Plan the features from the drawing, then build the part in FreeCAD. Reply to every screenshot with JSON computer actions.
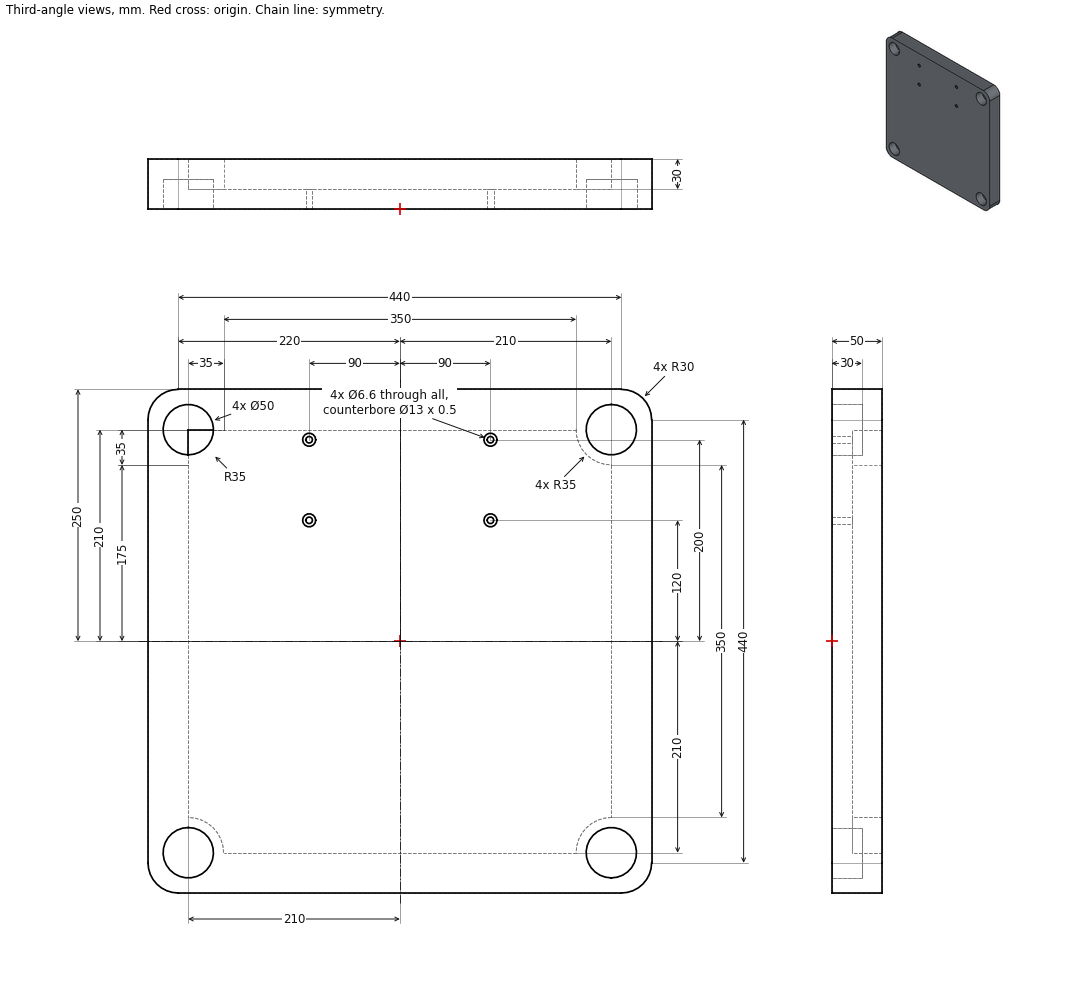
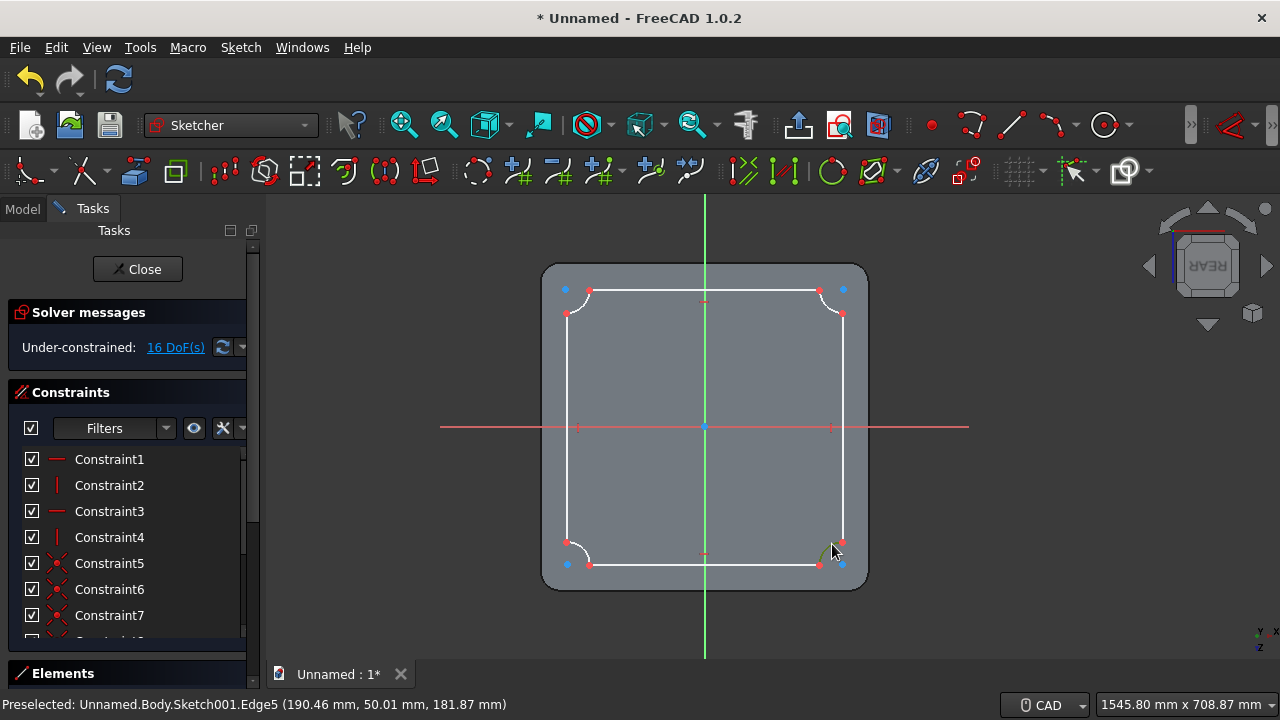
{"action": "scroll", "coordinate": [823, 301], "scroll_direction": "up", "scroll_amount": 2}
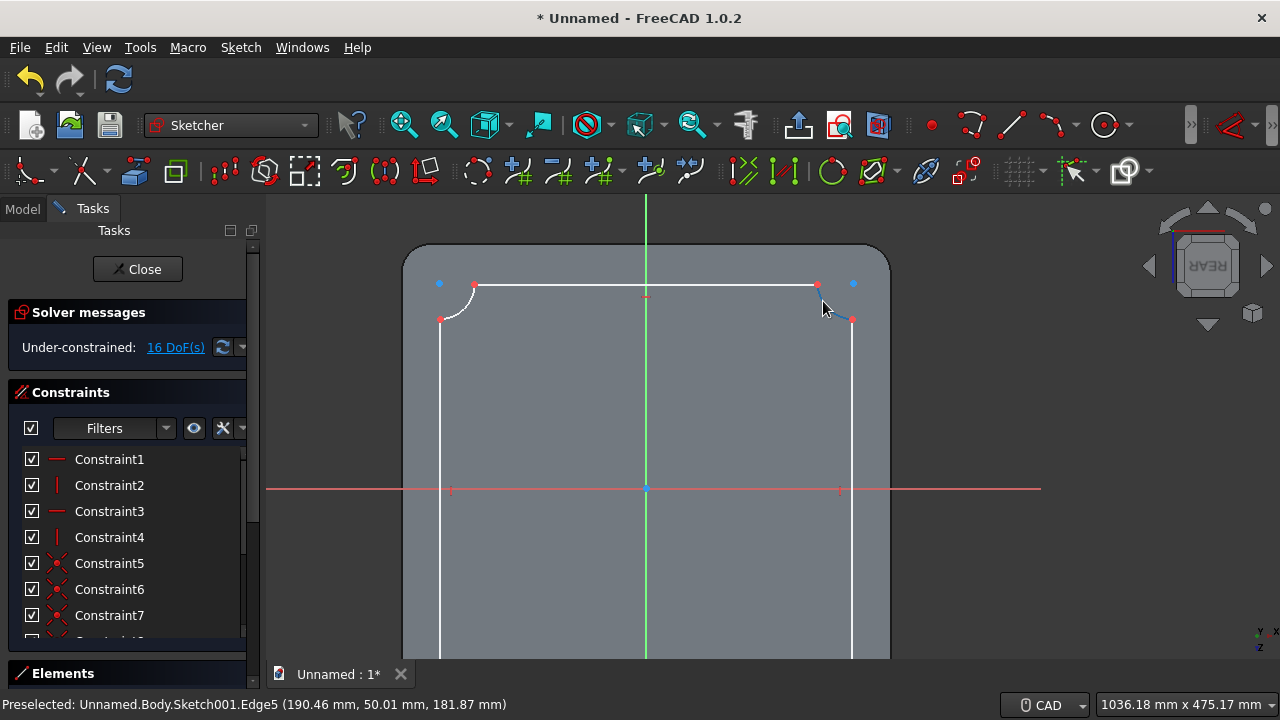
{"action": "left_click", "coordinate": [822, 300]}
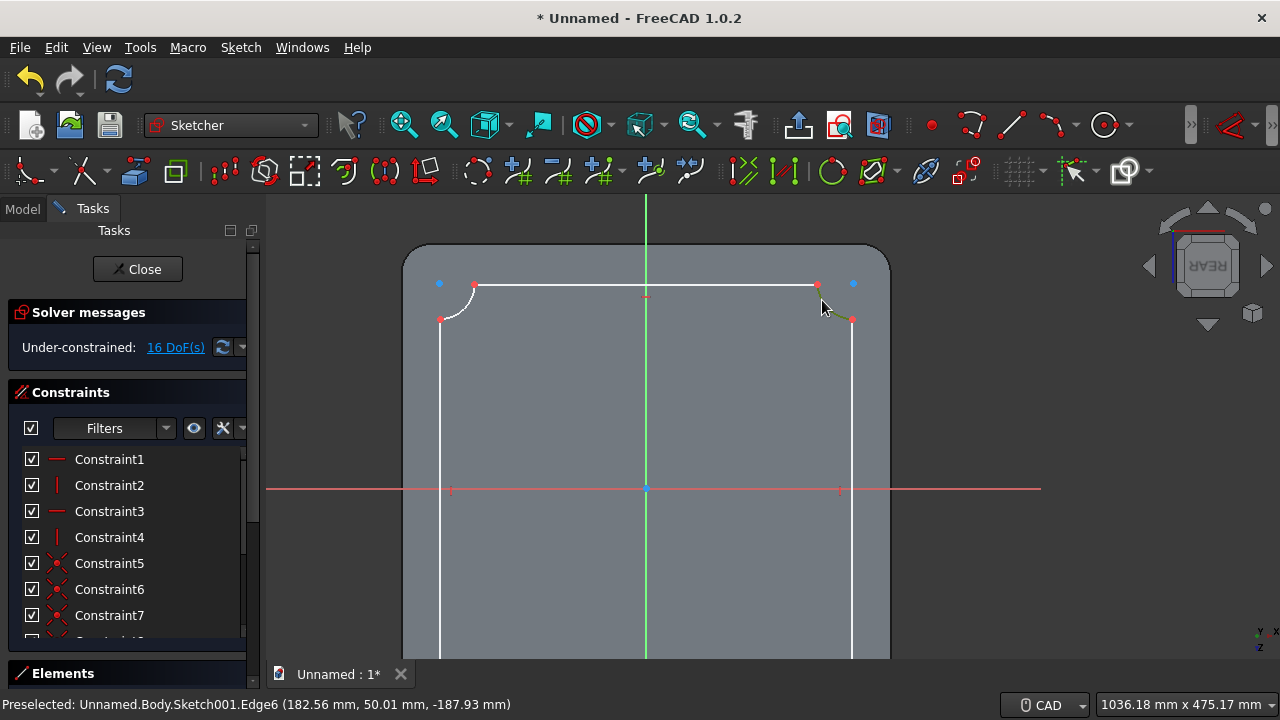
{"action": "left_click", "coordinate": [456, 315]}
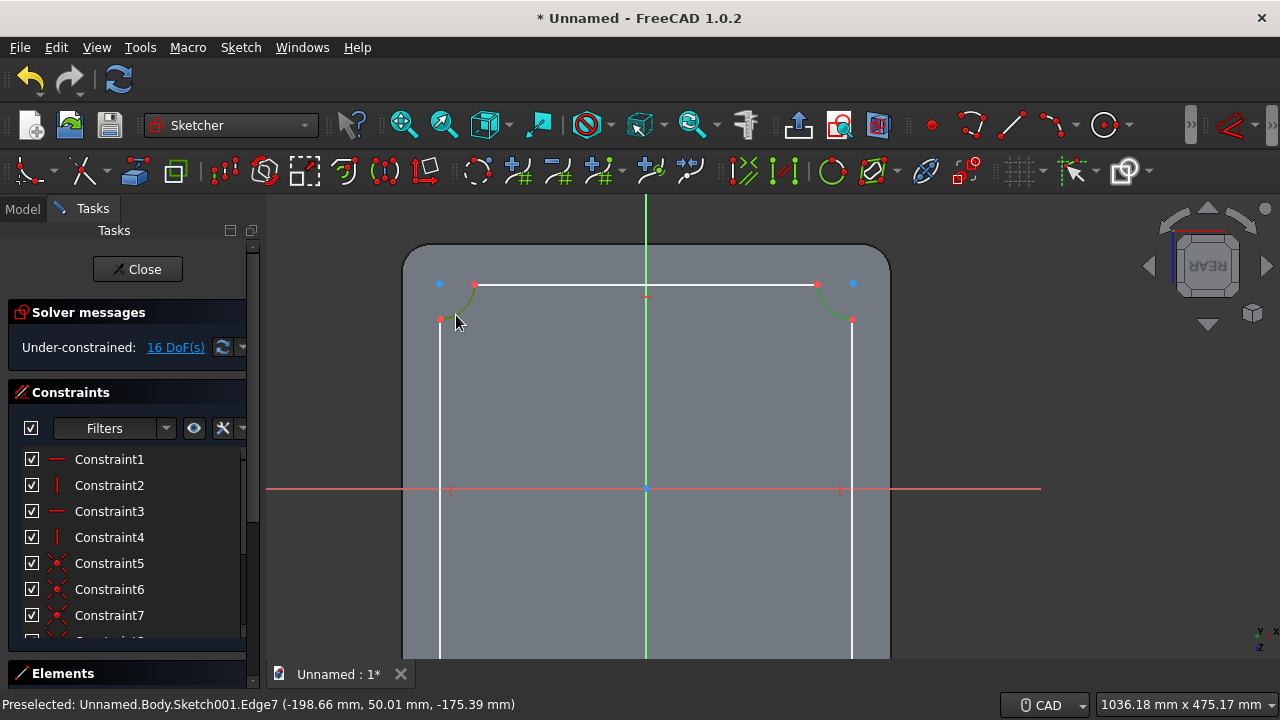
{"action": "scroll", "coordinate": [823, 300], "scroll_direction": "down", "scroll_amount": 2}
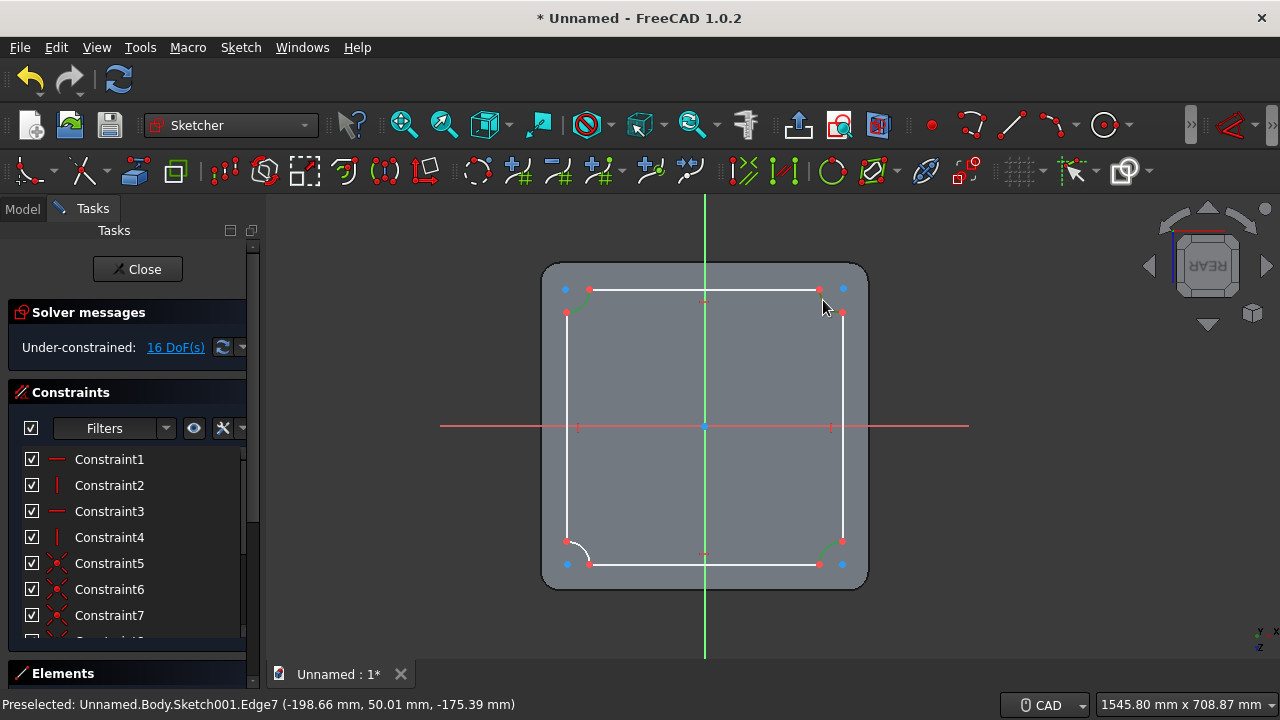
{"action": "scroll", "coordinate": [587, 554], "scroll_direction": "up", "scroll_amount": 2}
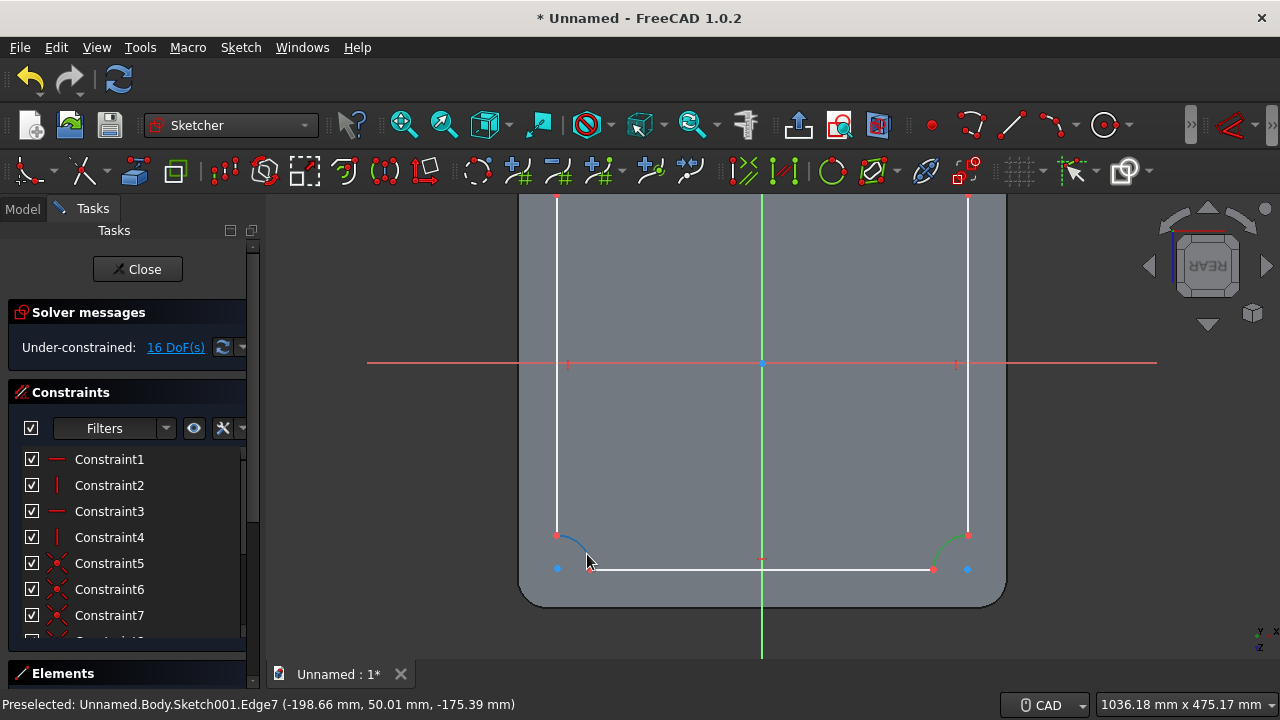
{"action": "left_click", "coordinate": [587, 554]}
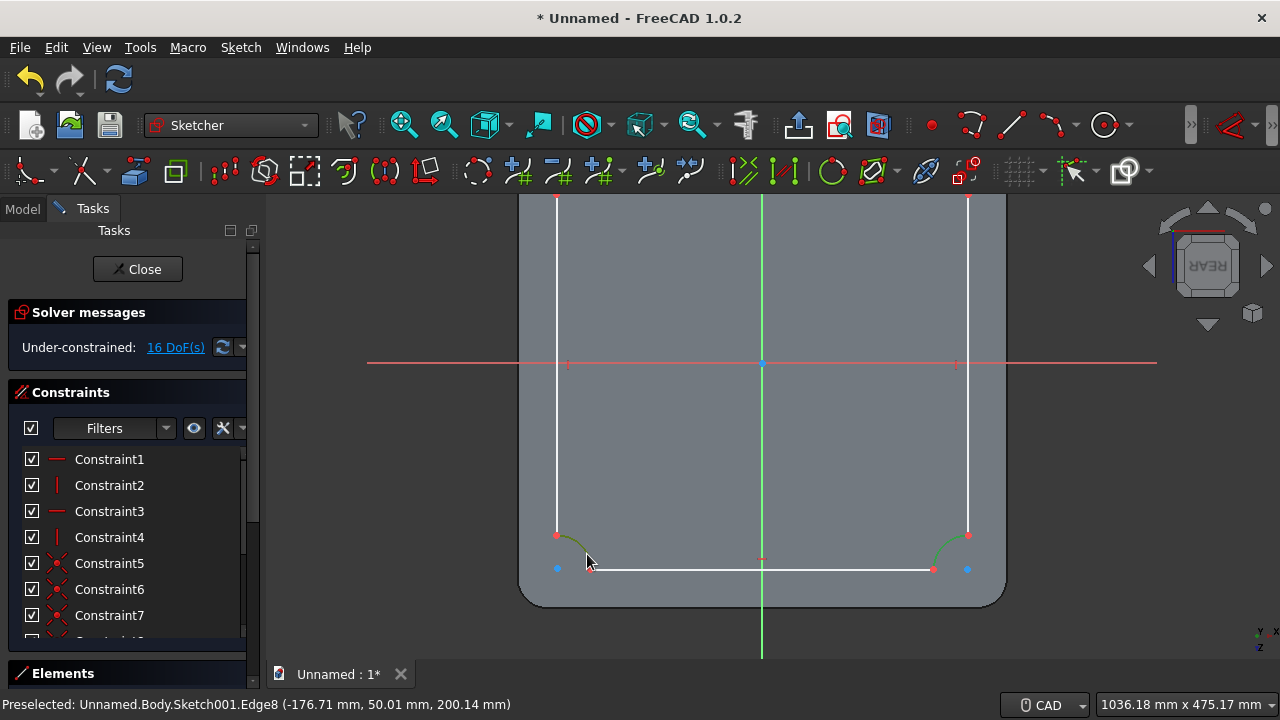
{"action": "key", "text": "e"}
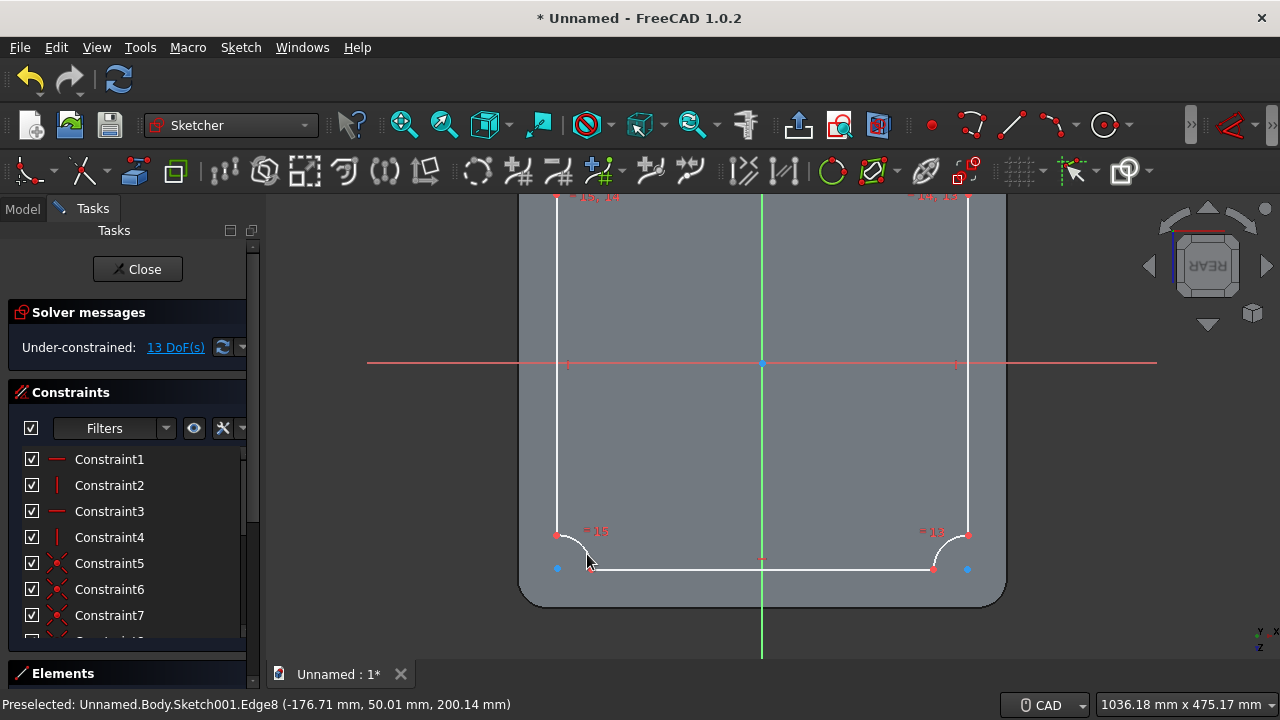
{"action": "left_click", "coordinate": [968, 569]}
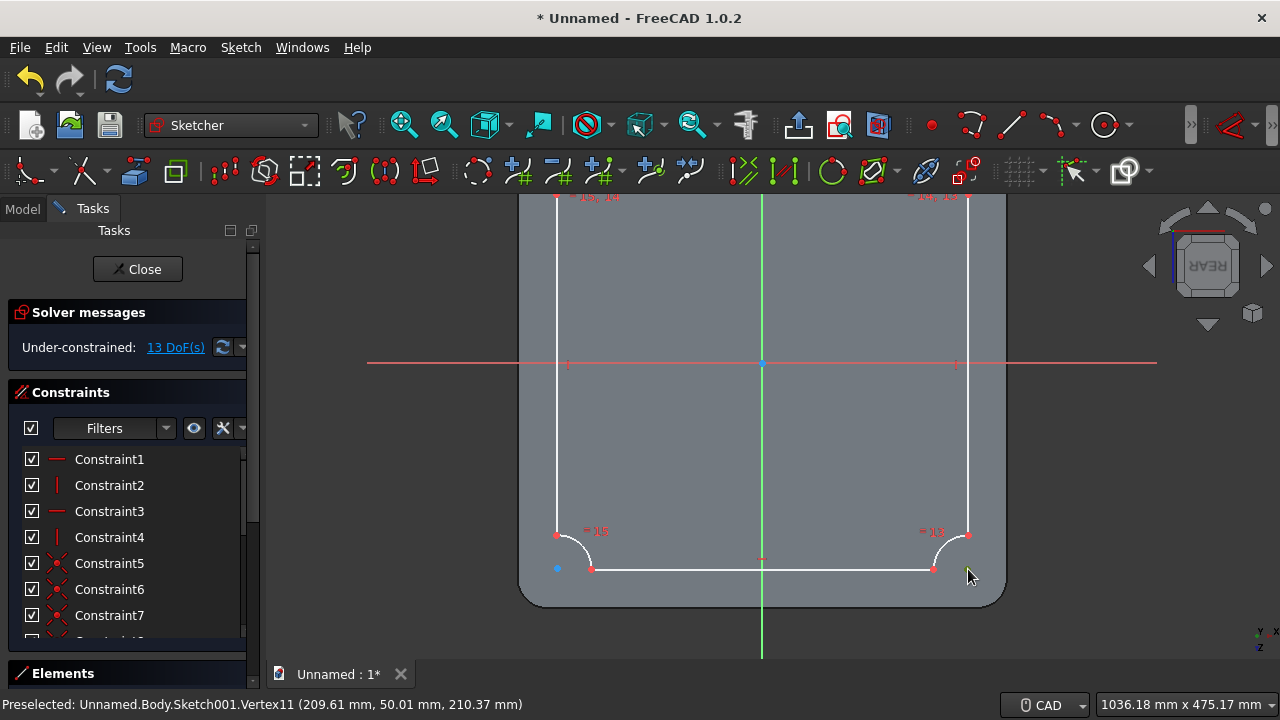
{"action": "scroll", "coordinate": [587, 555], "scroll_direction": "down", "scroll_amount": 2}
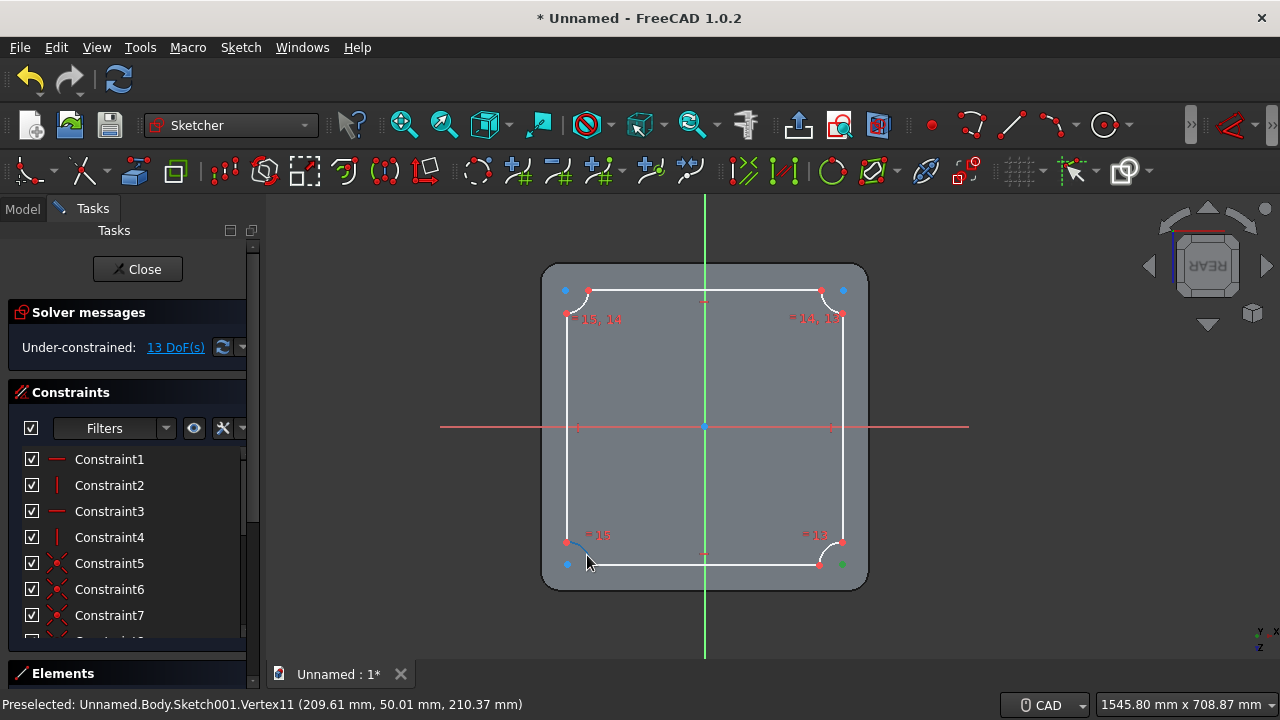
{"action": "left_click", "coordinate": [844, 291]}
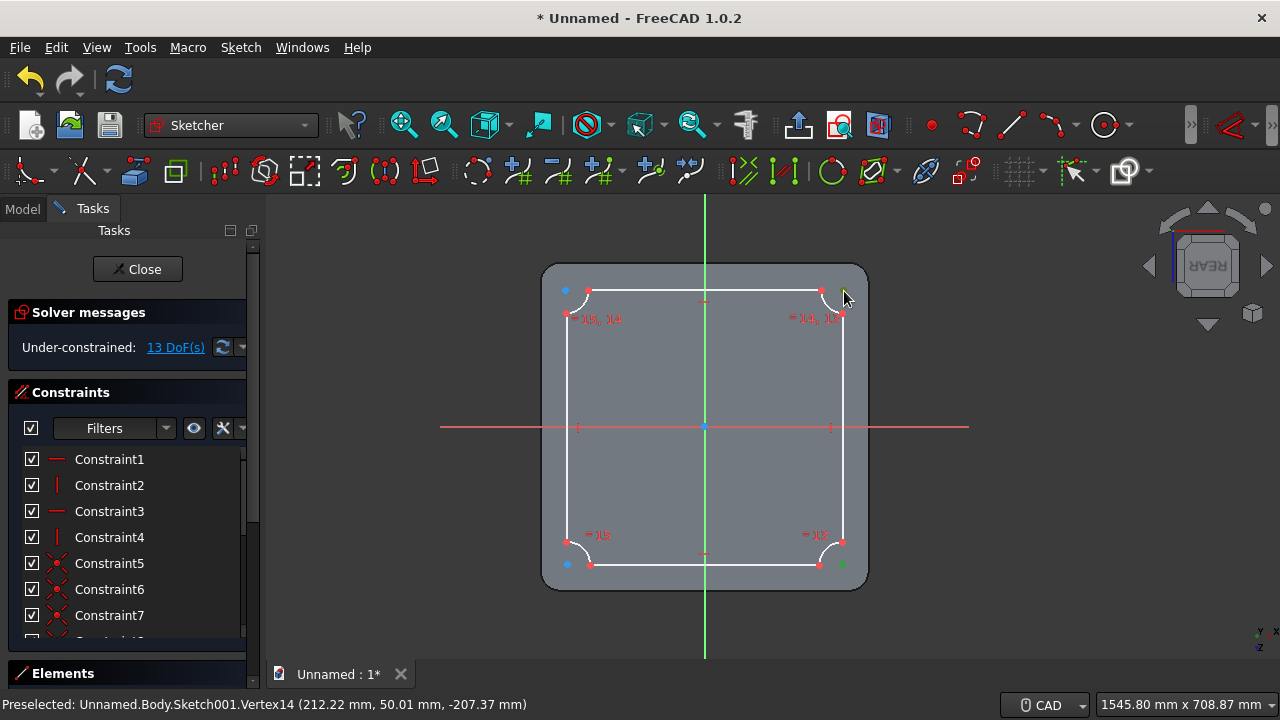
{"action": "left_click", "coordinate": [470, 427]}